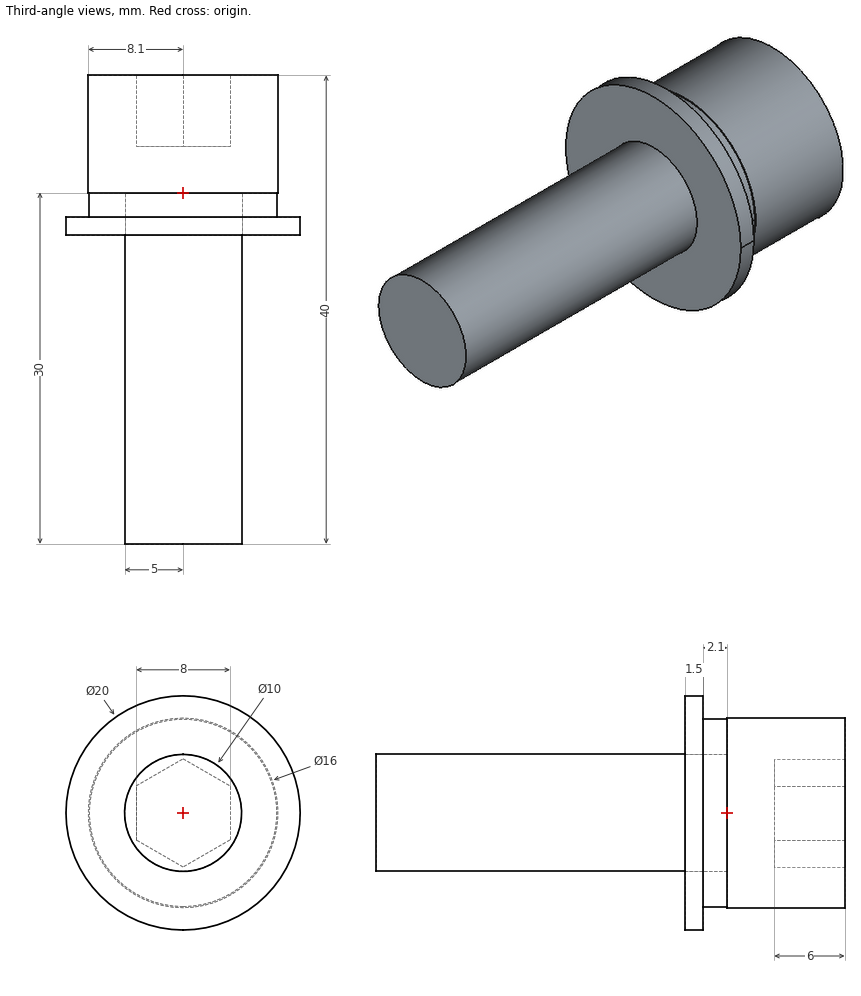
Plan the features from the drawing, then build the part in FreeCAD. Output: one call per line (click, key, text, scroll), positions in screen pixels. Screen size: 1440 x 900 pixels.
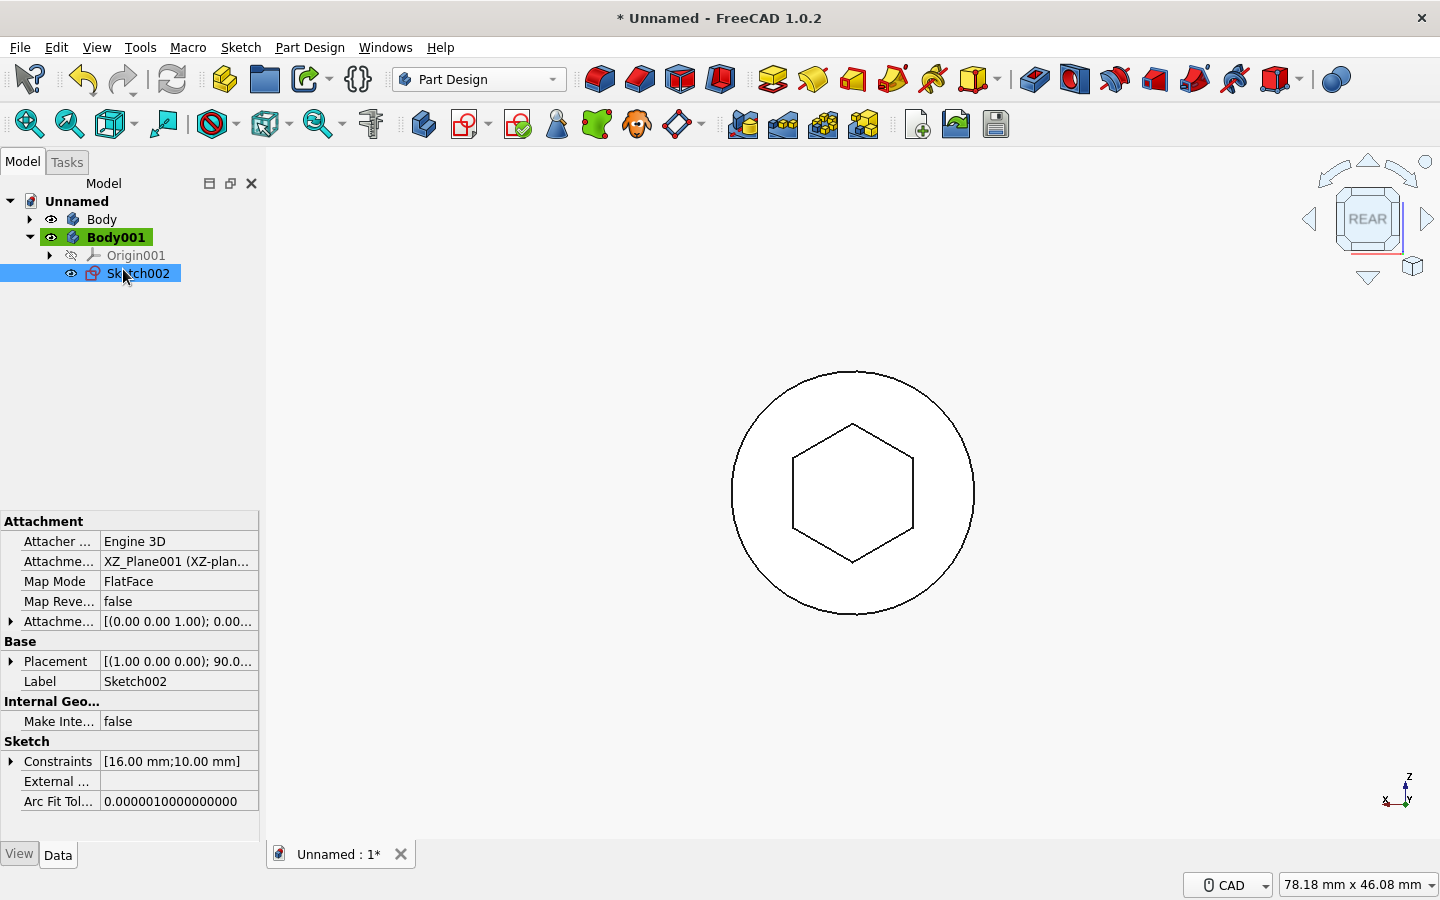
click(774, 80)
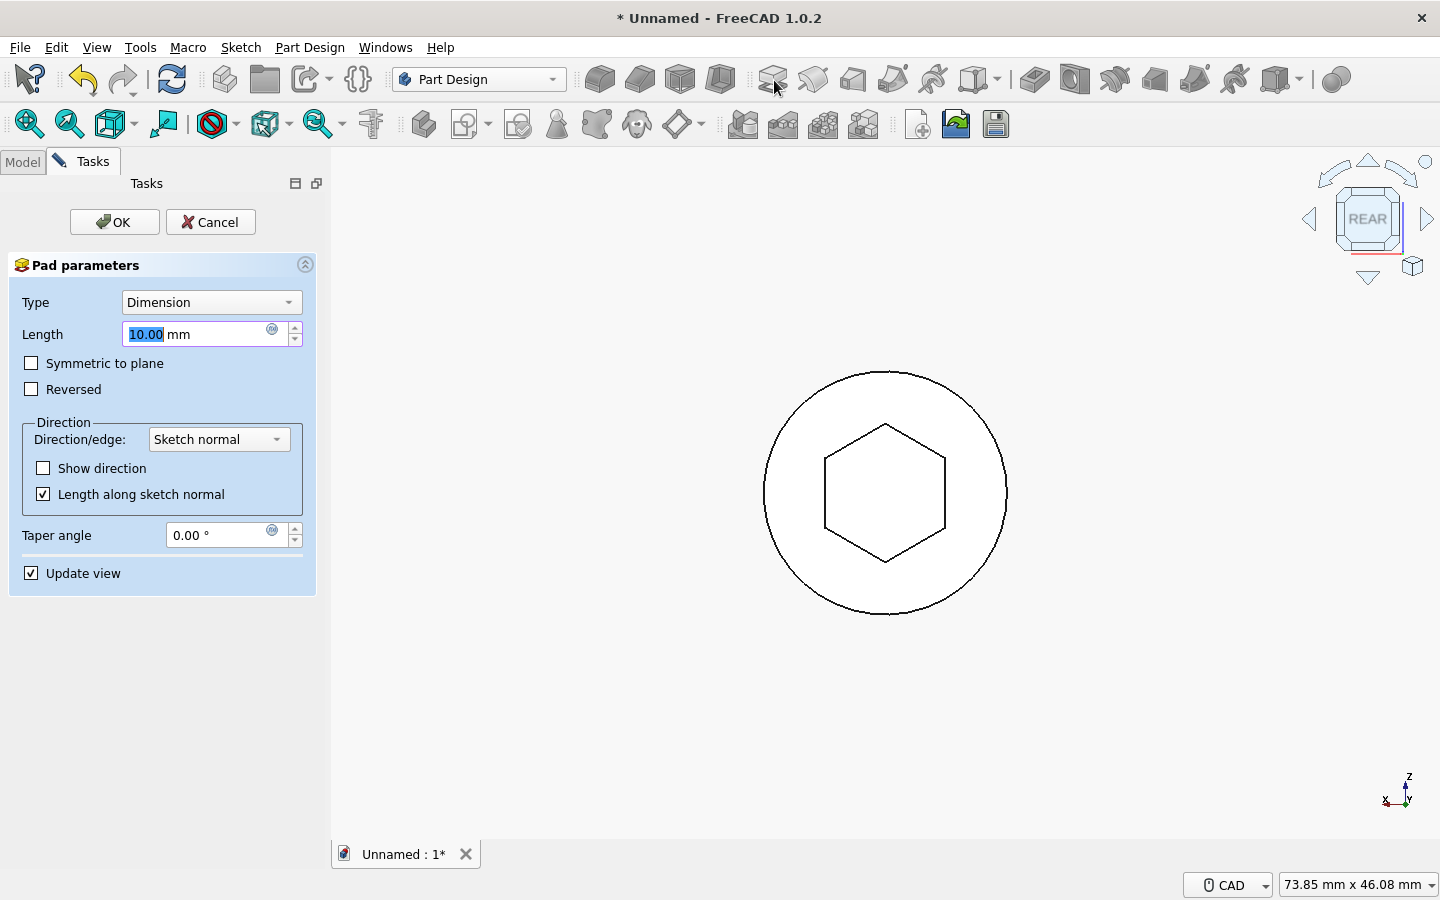
text(2.1)
key(Tab)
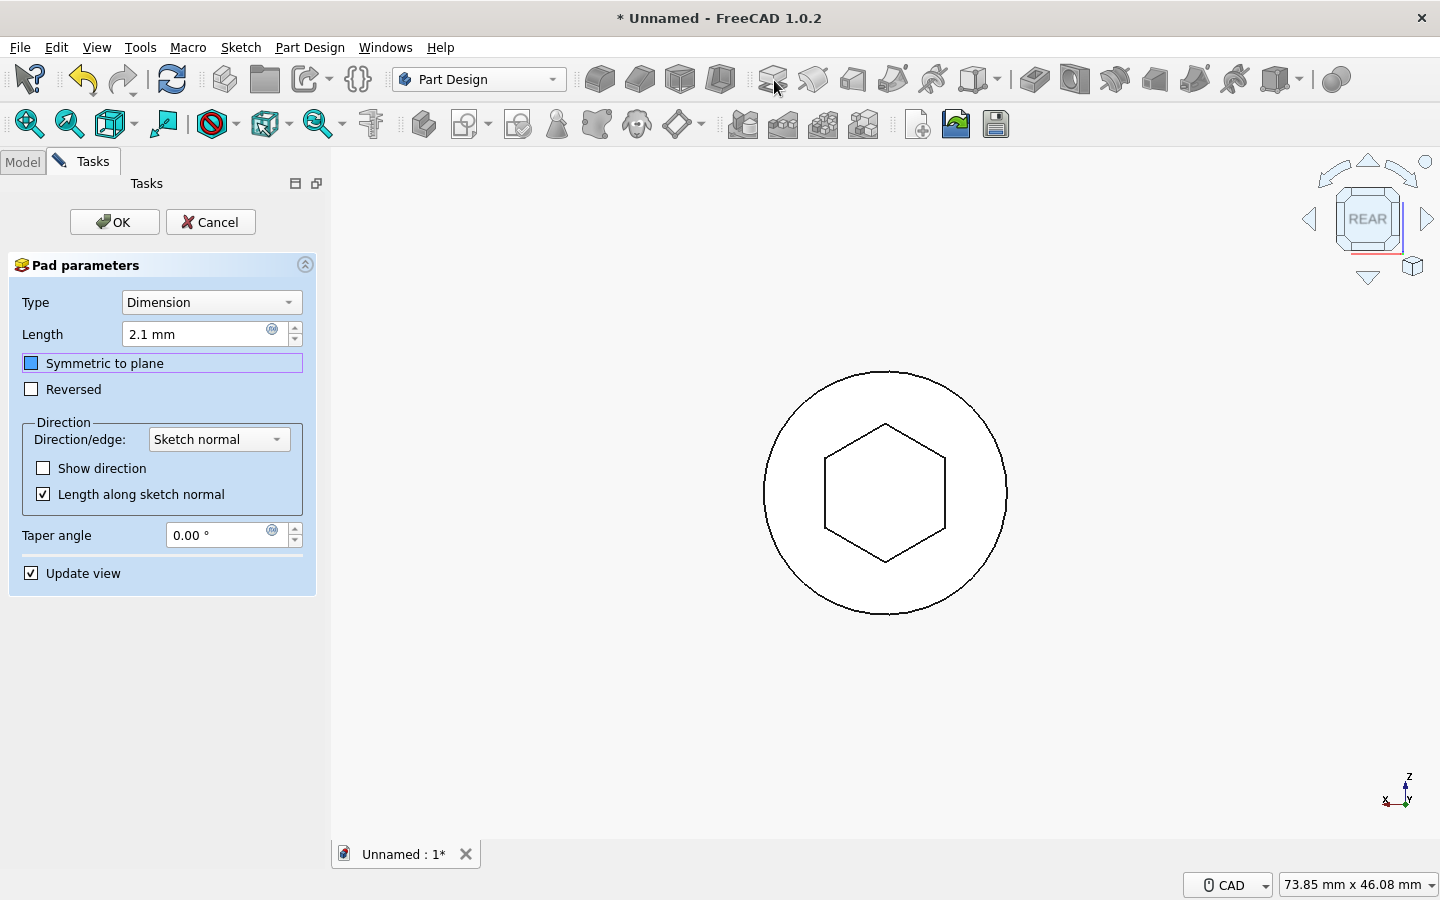
click(115, 222)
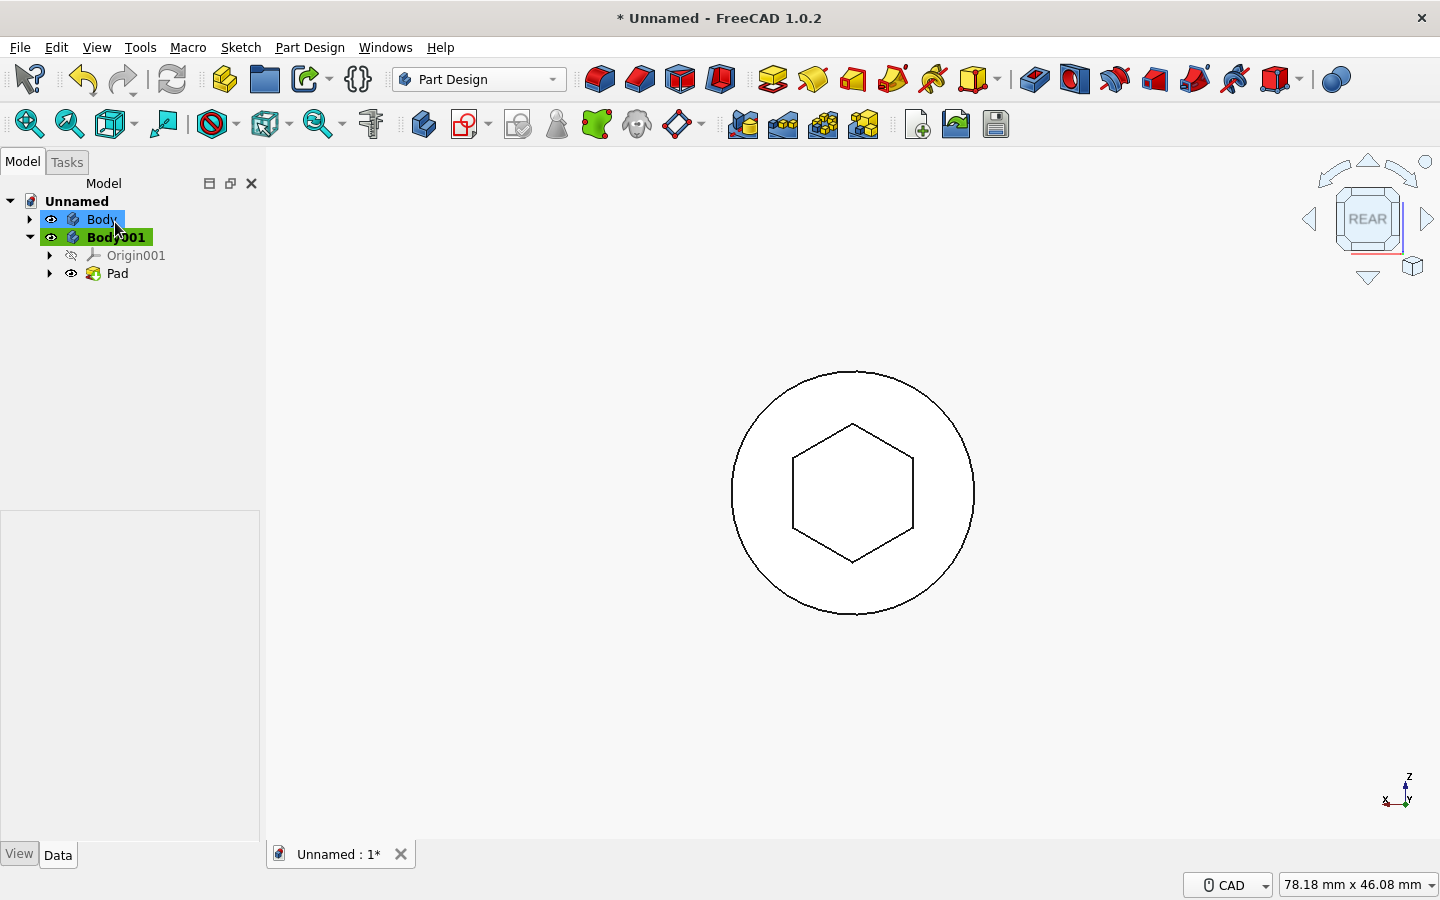
click(30, 124)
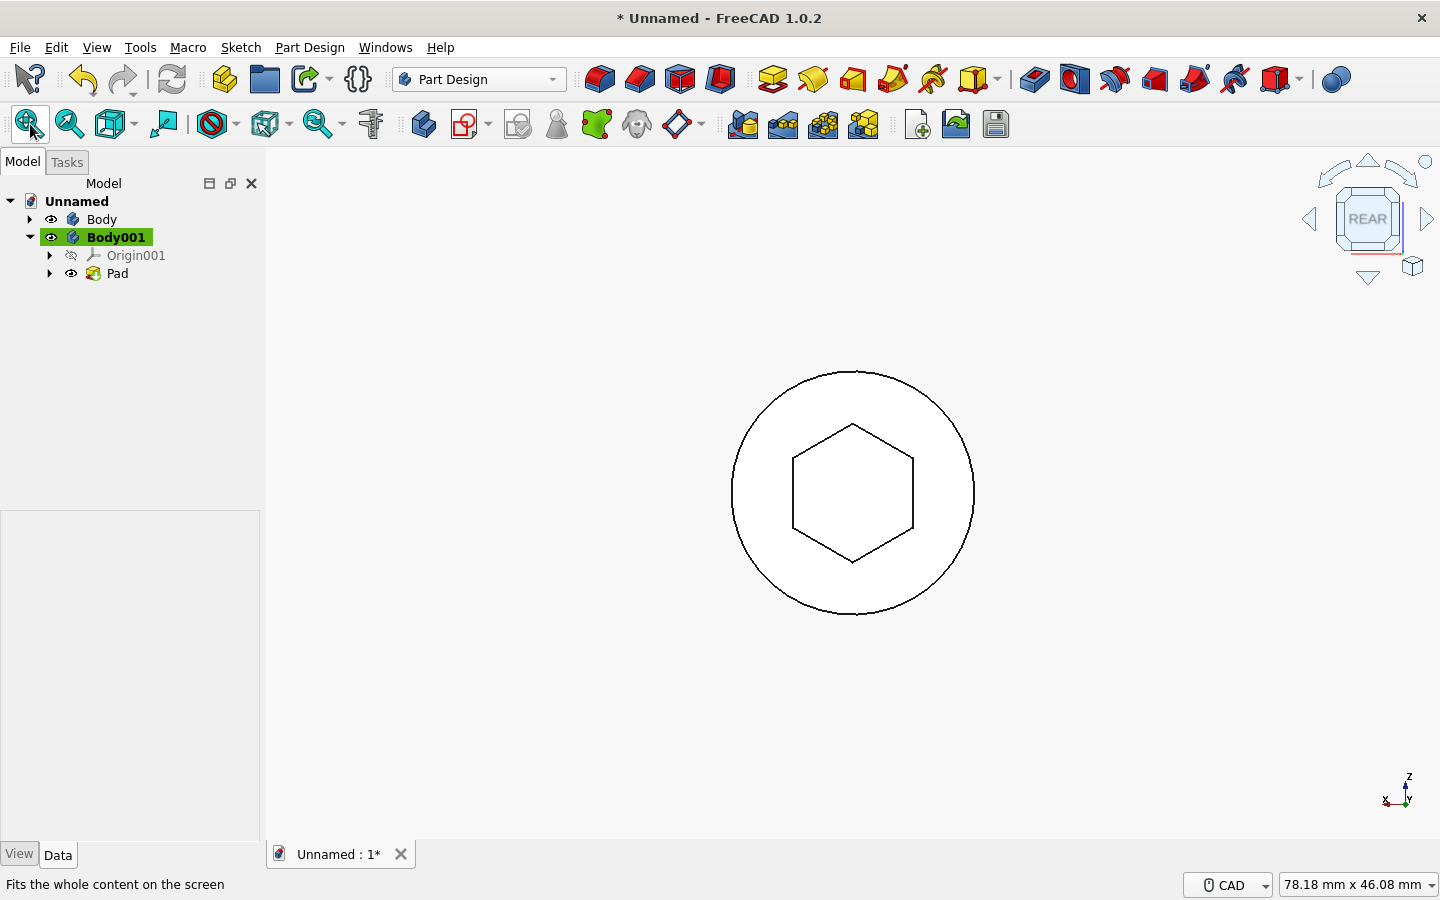
click(424, 124)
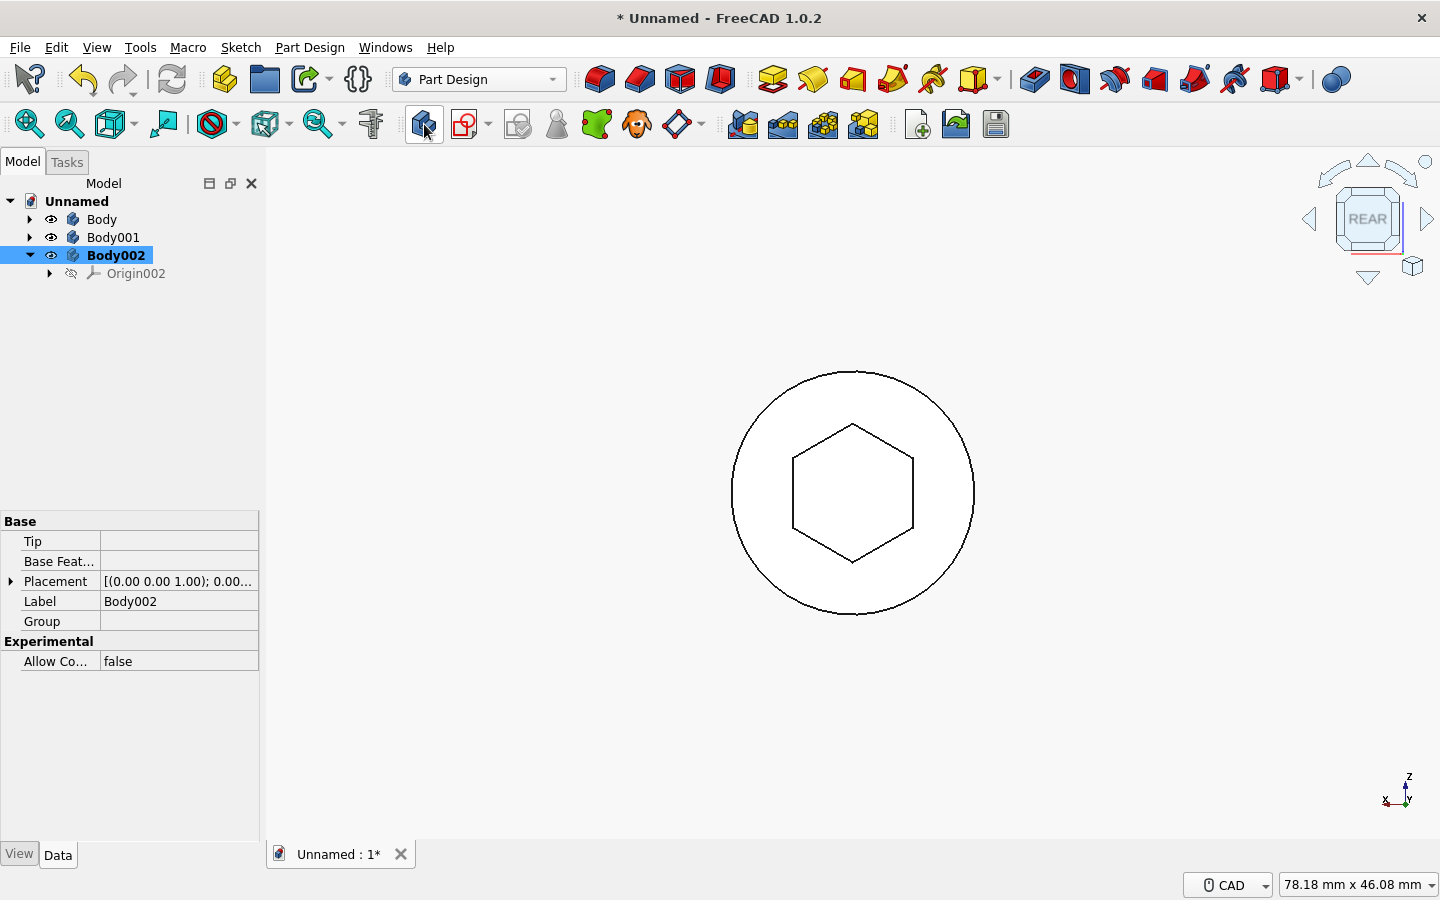
click(50, 273)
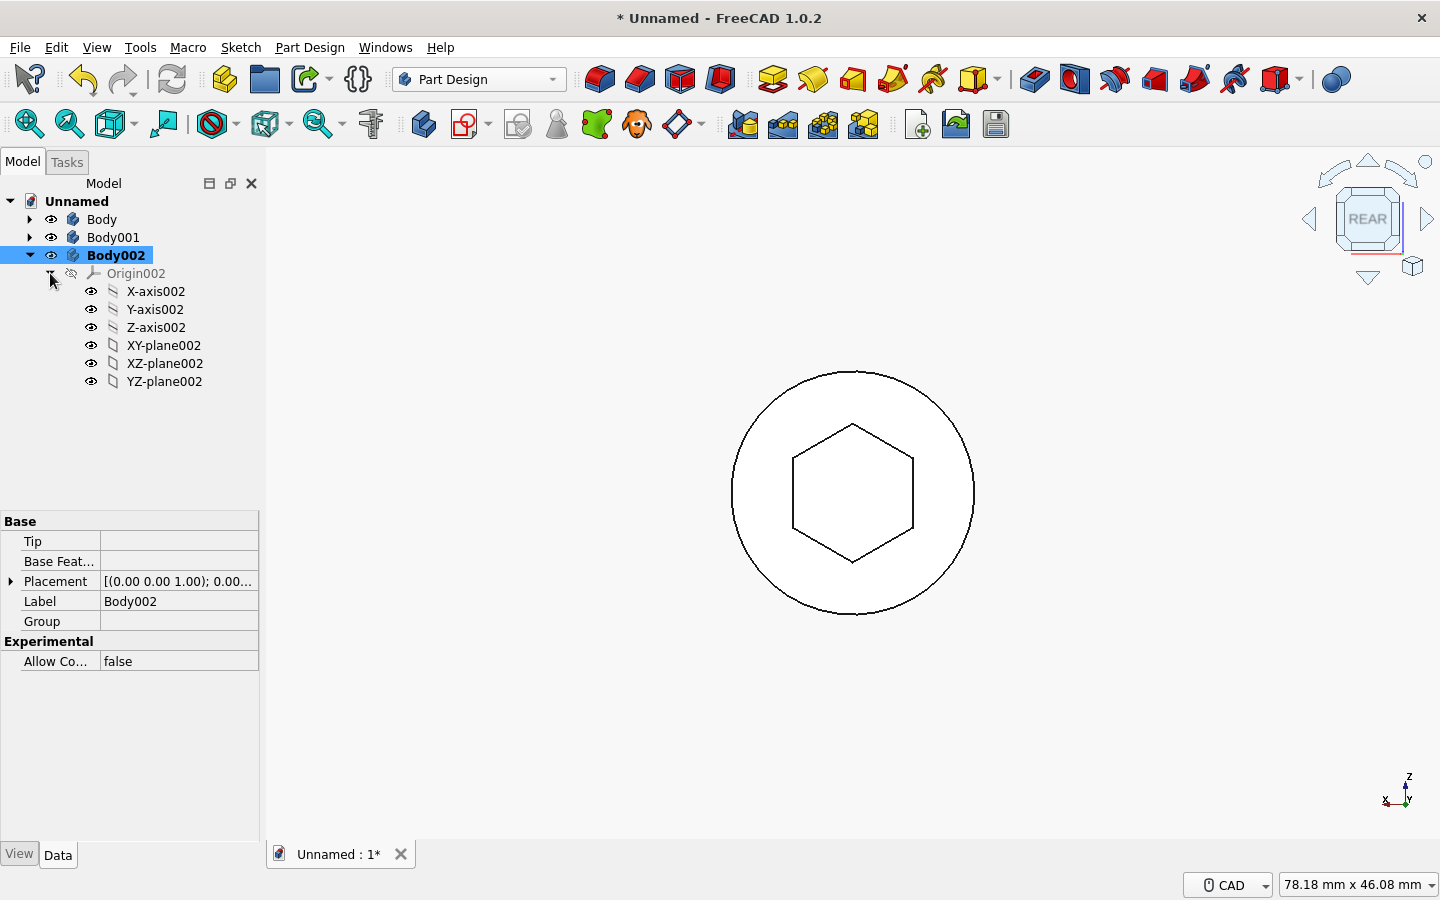
click(136, 363)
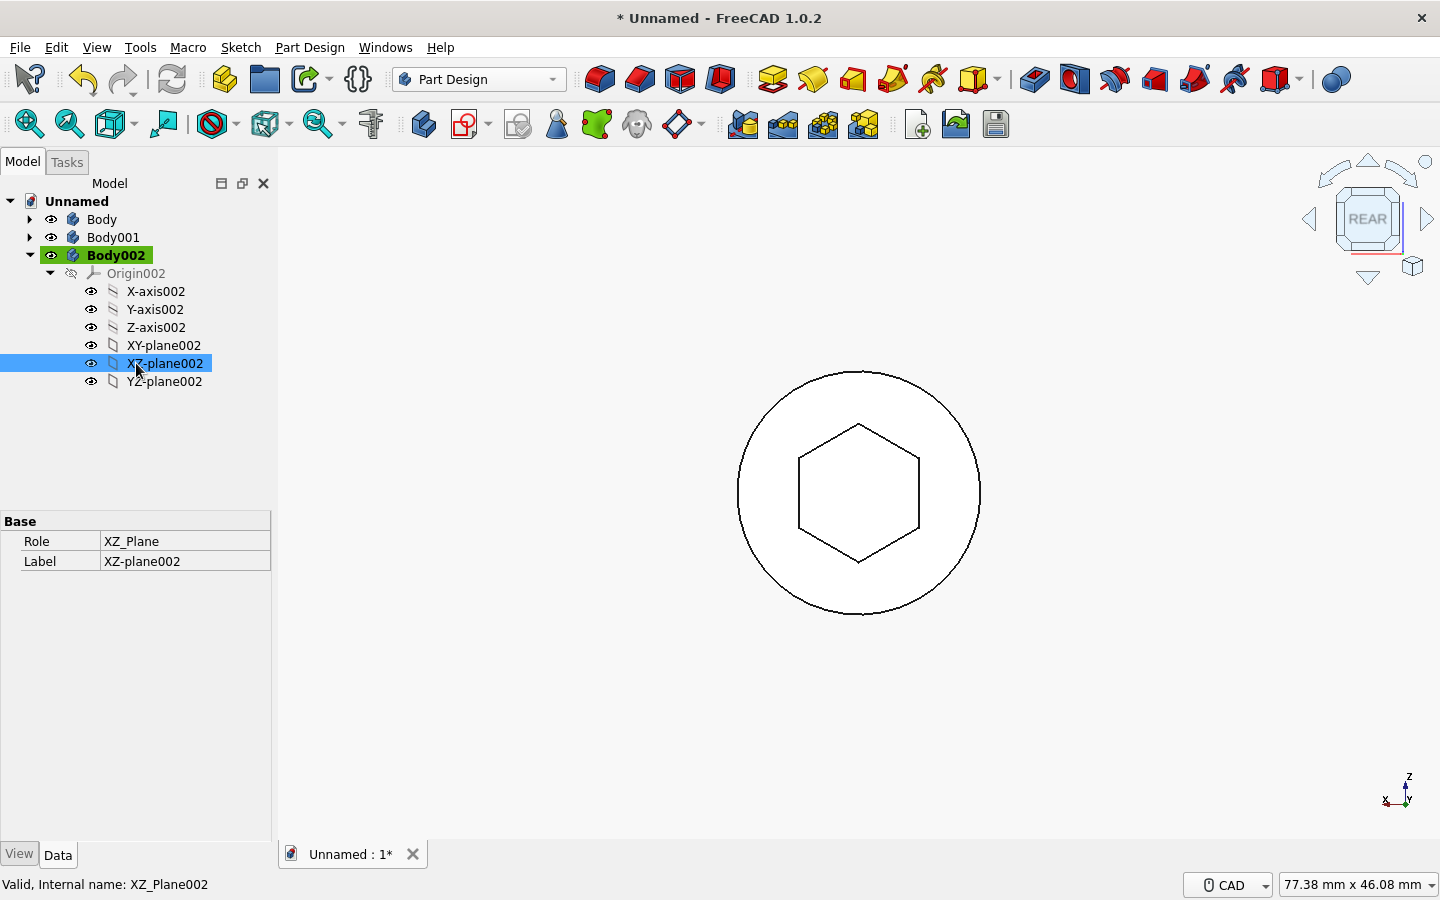
click(678, 124)